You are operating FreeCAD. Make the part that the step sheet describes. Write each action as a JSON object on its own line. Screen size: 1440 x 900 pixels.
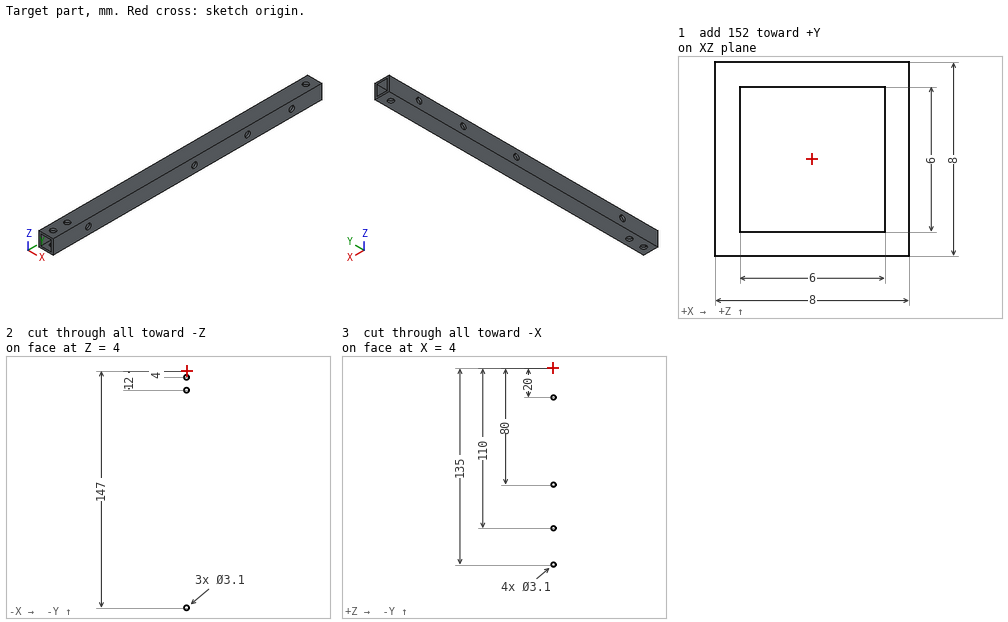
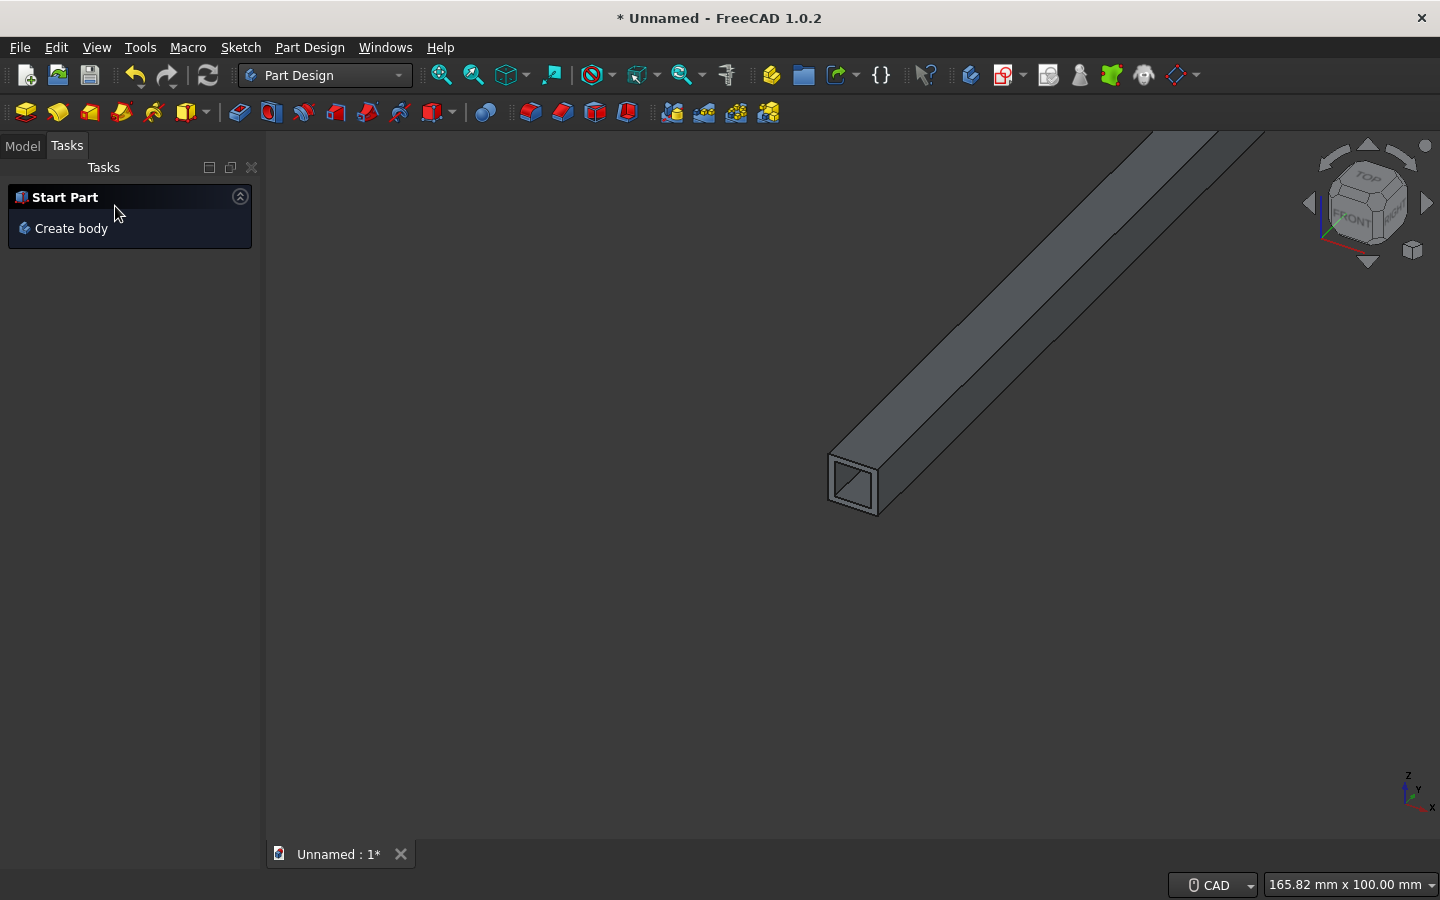
{"action": "left_click", "coordinate": [442, 76]}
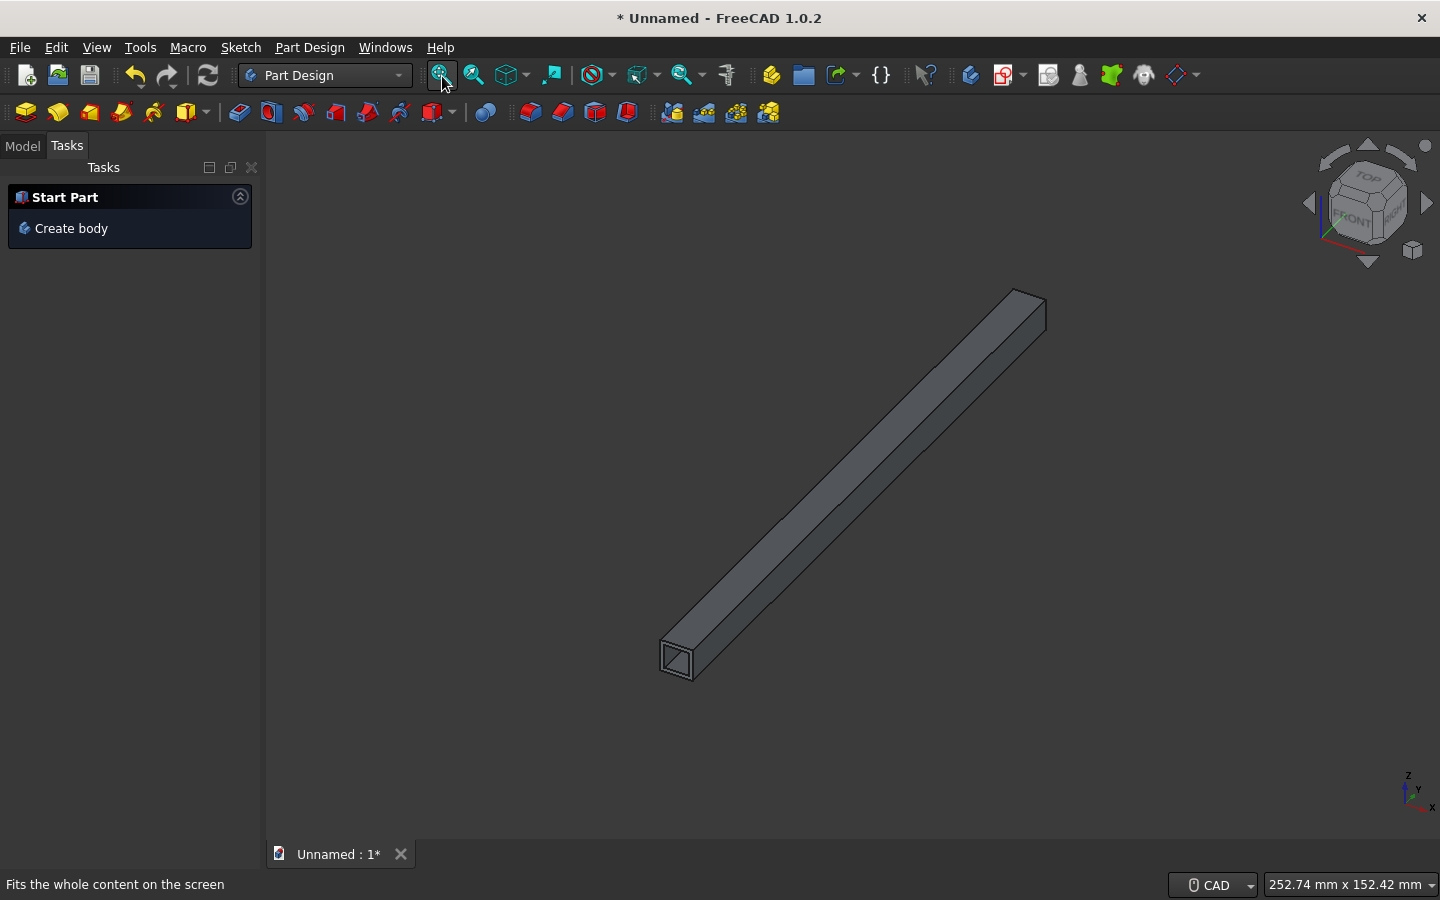
{"action": "left_click", "coordinate": [1004, 318]}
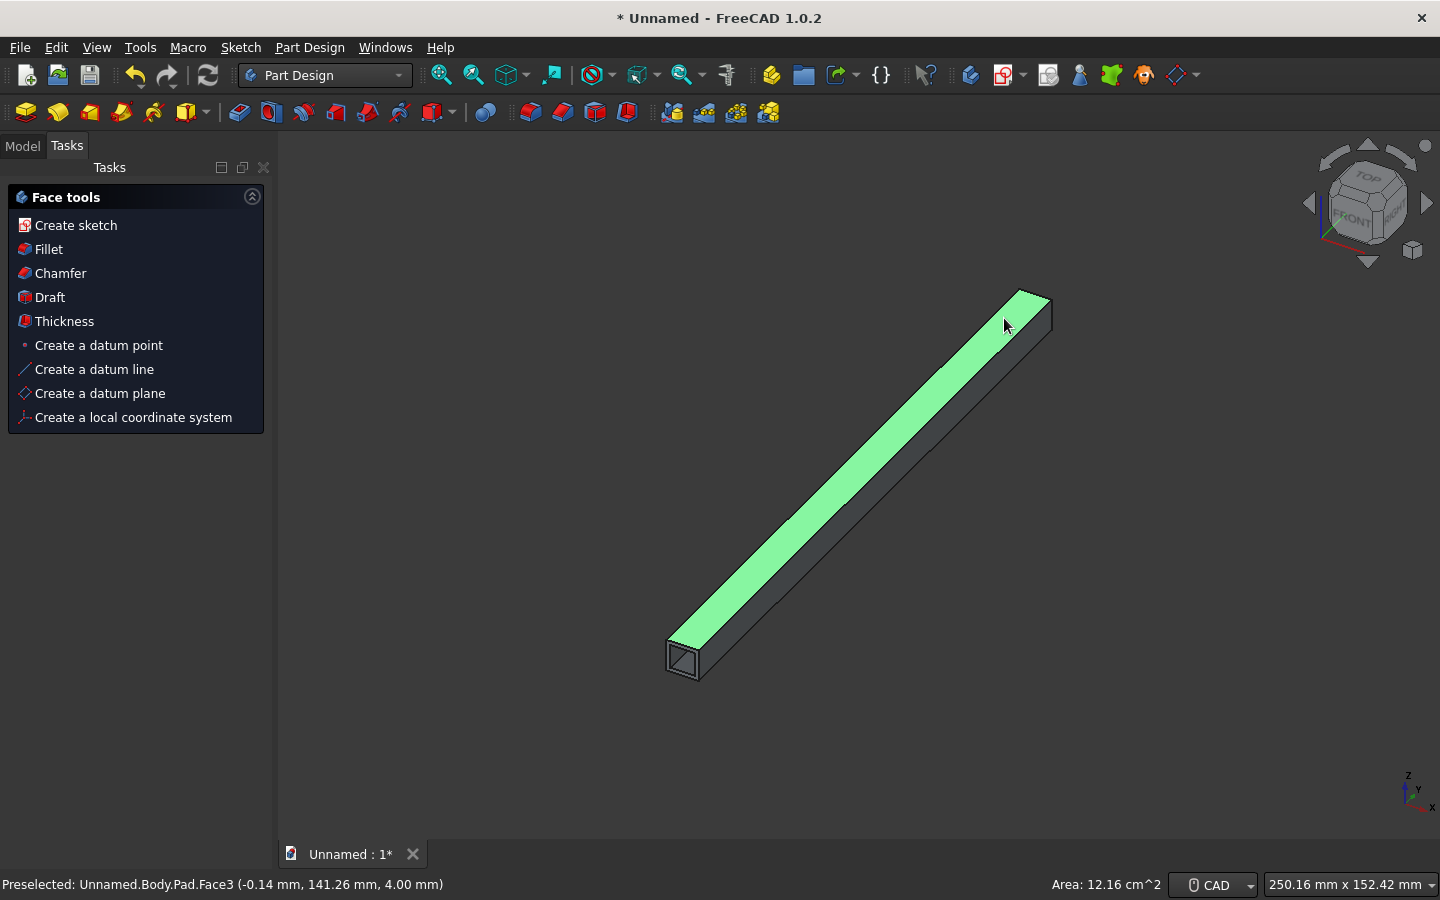
{"action": "left_click", "coordinate": [1004, 76]}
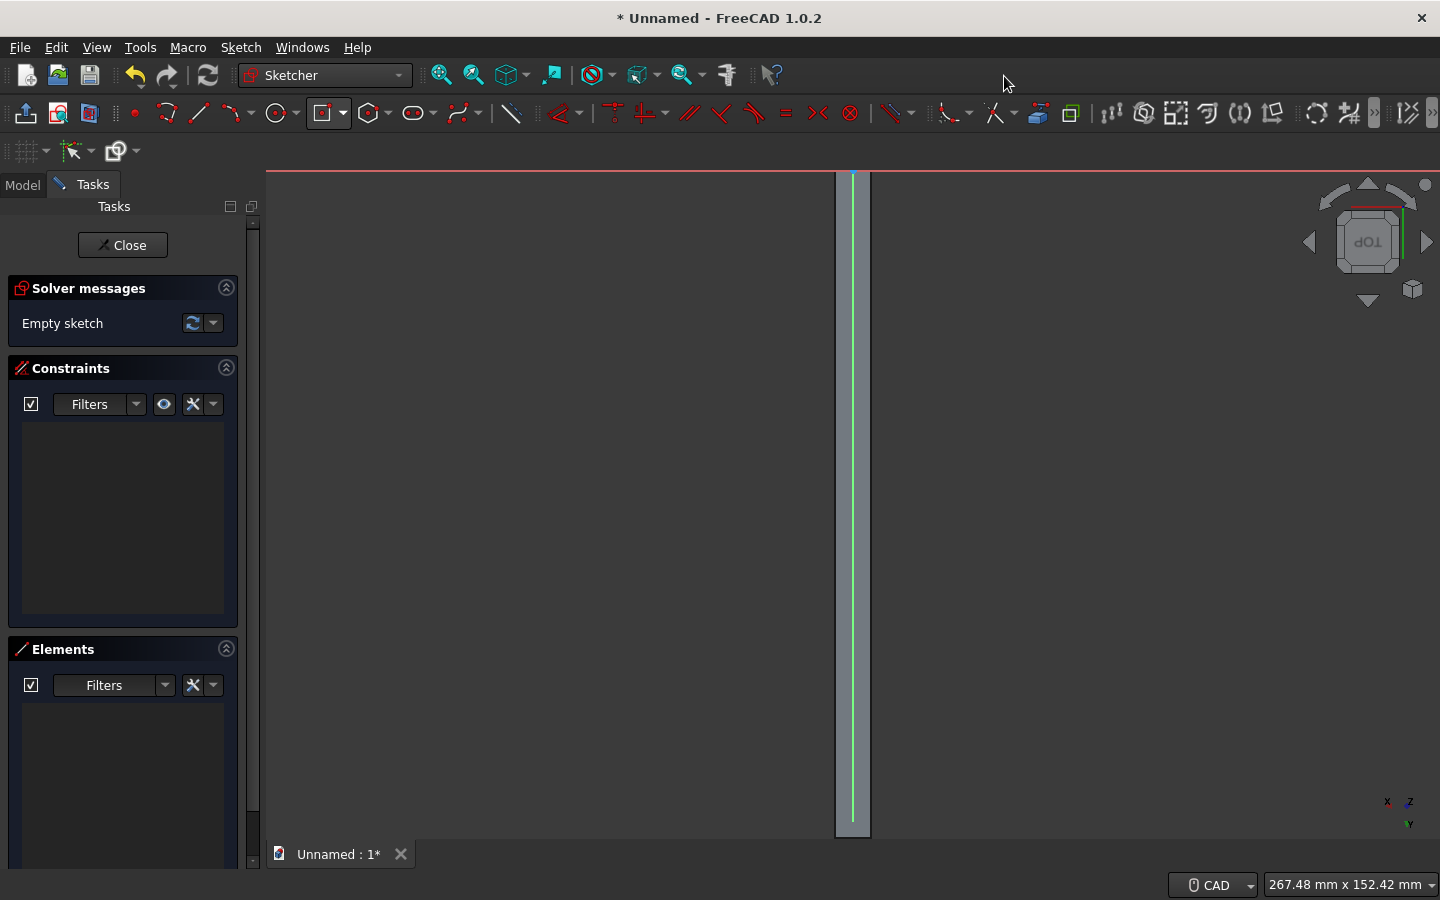
{"action": "scroll", "coordinate": [645, 520], "scroll_direction": "down", "scroll_amount": 2}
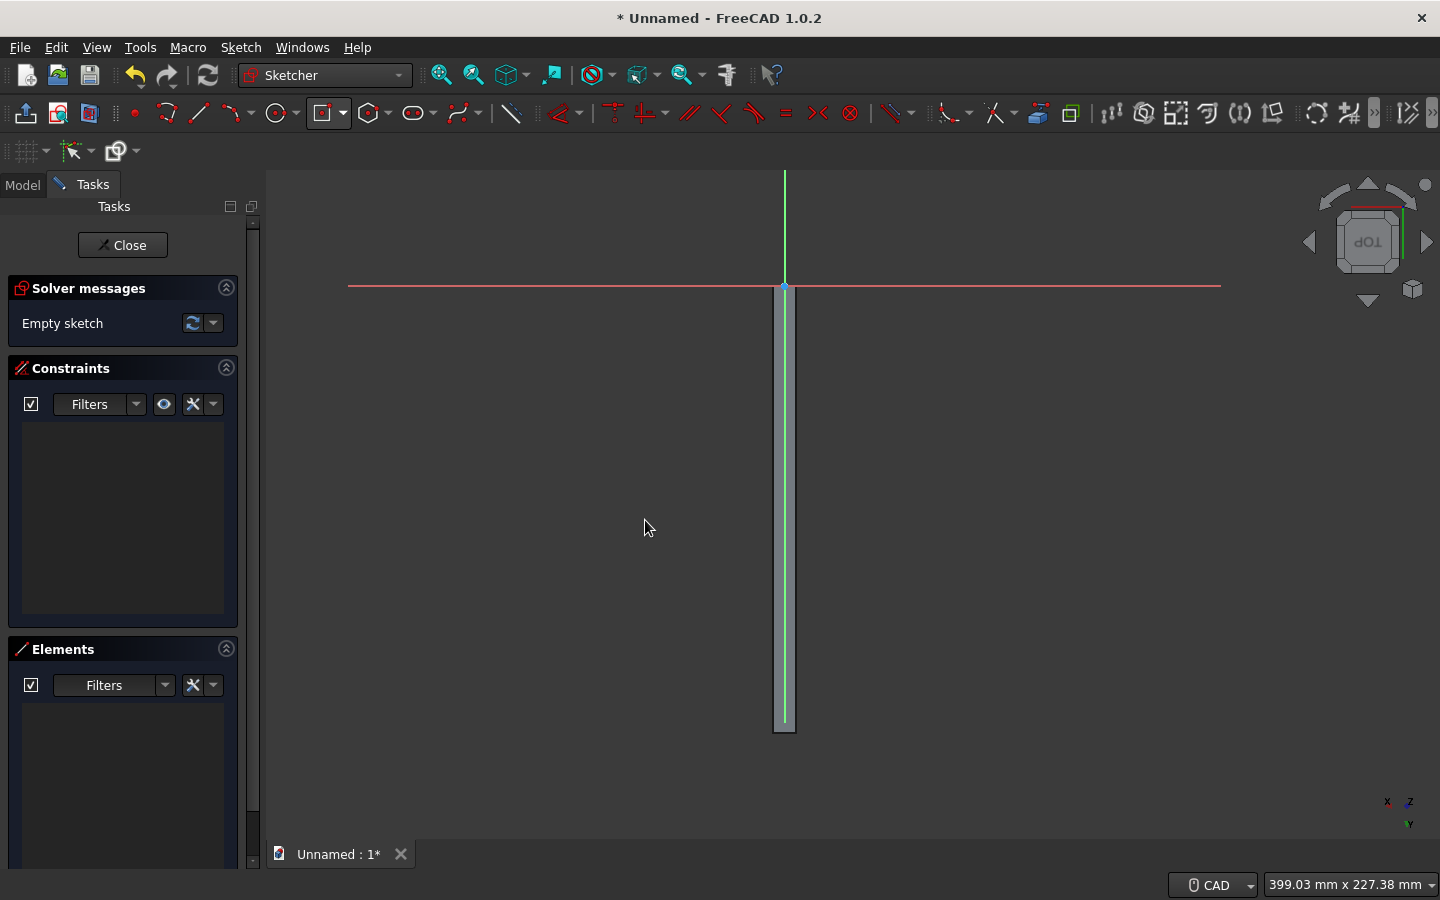
{"action": "left_click", "coordinate": [276, 114]}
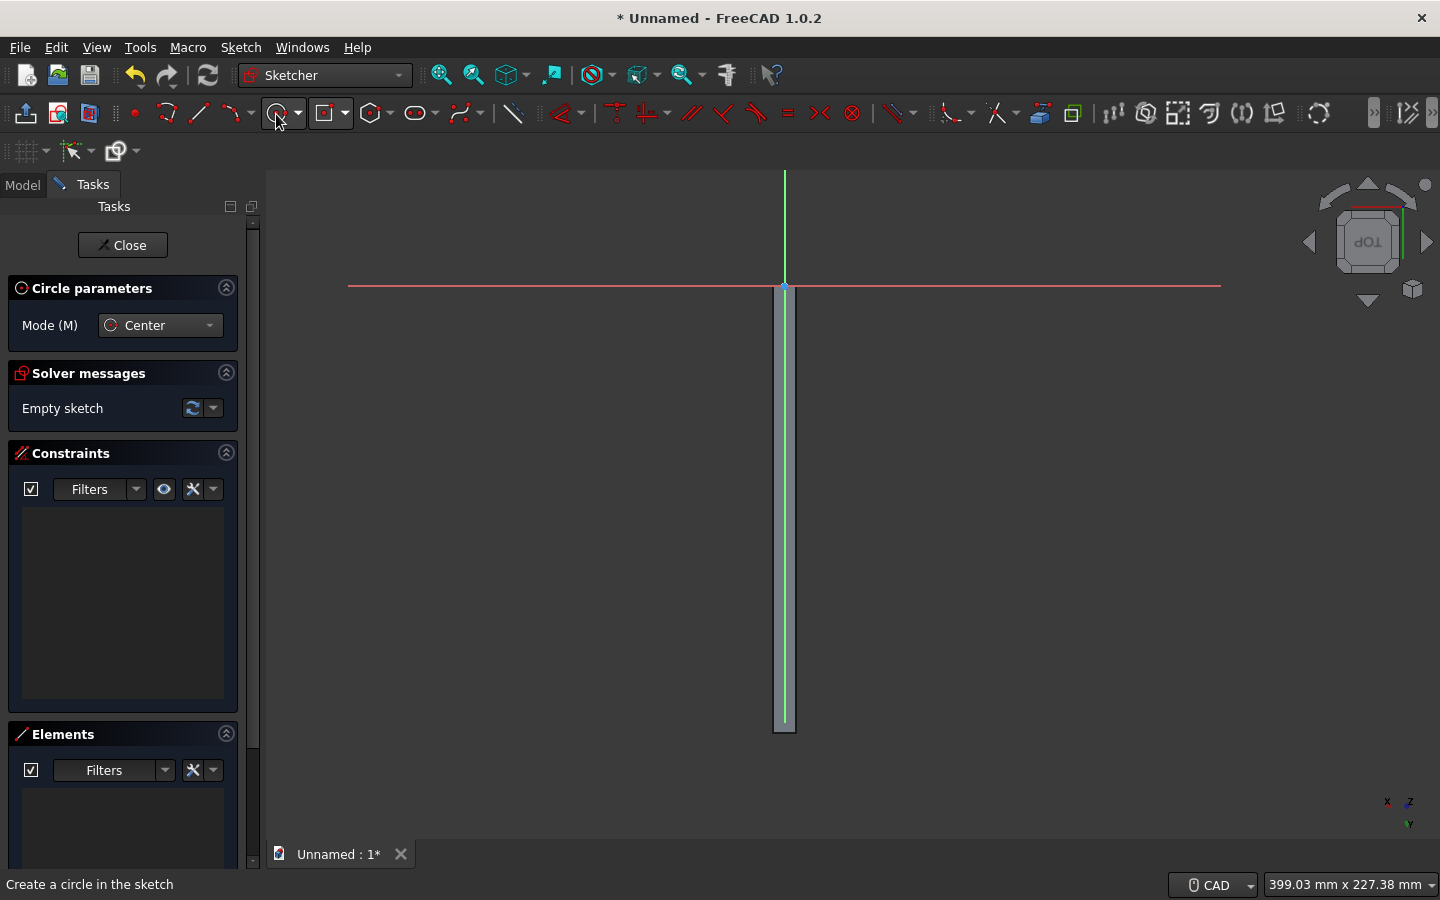
{"action": "scroll", "coordinate": [785, 719], "scroll_direction": "up", "scroll_amount": 9}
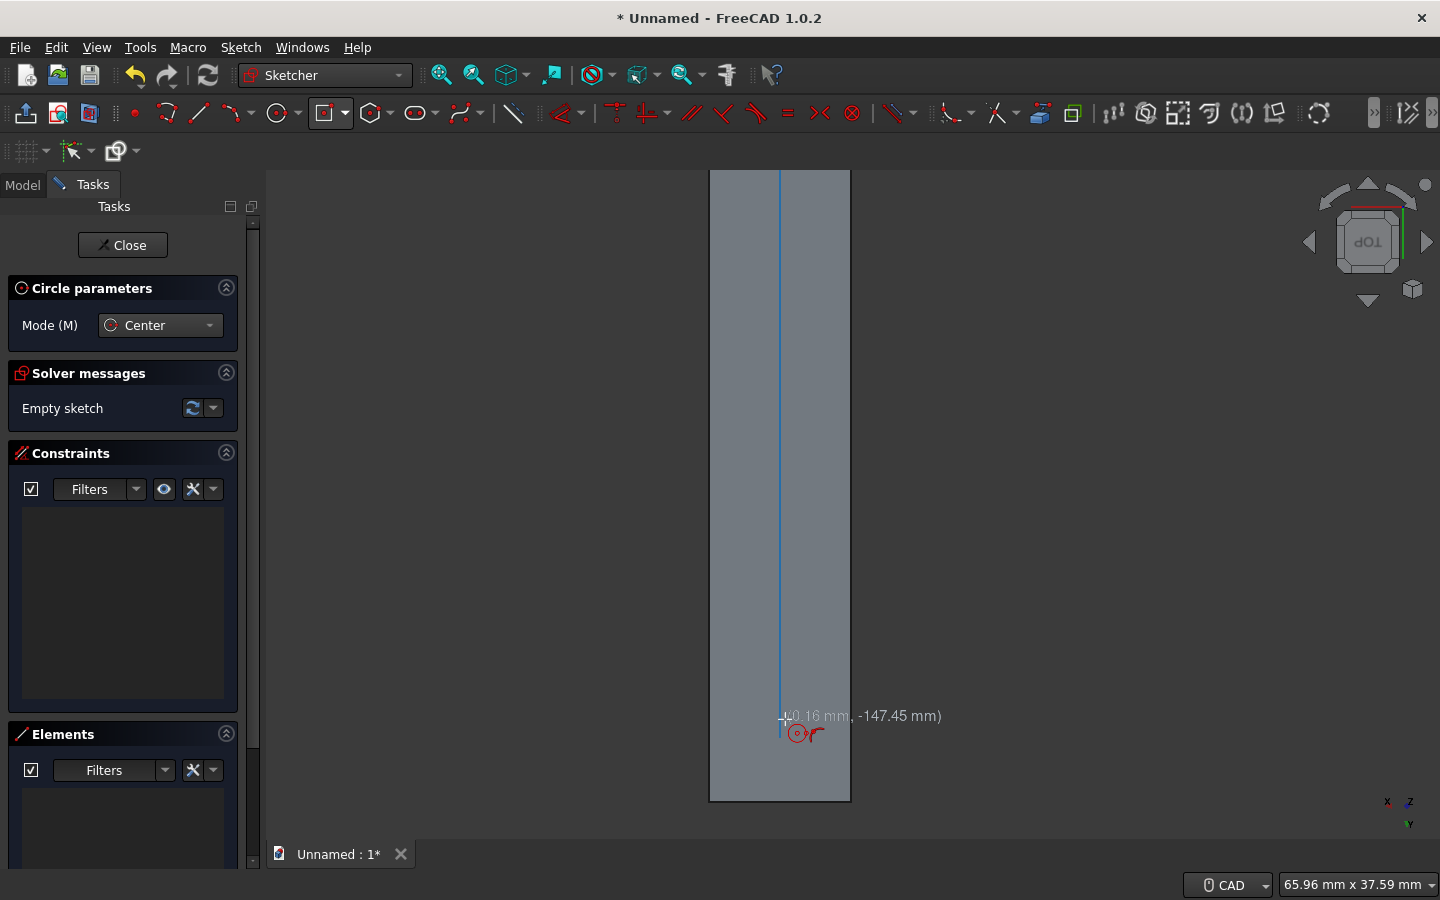
{"action": "scroll", "coordinate": [785, 720], "scroll_direction": "down", "scroll_amount": 9}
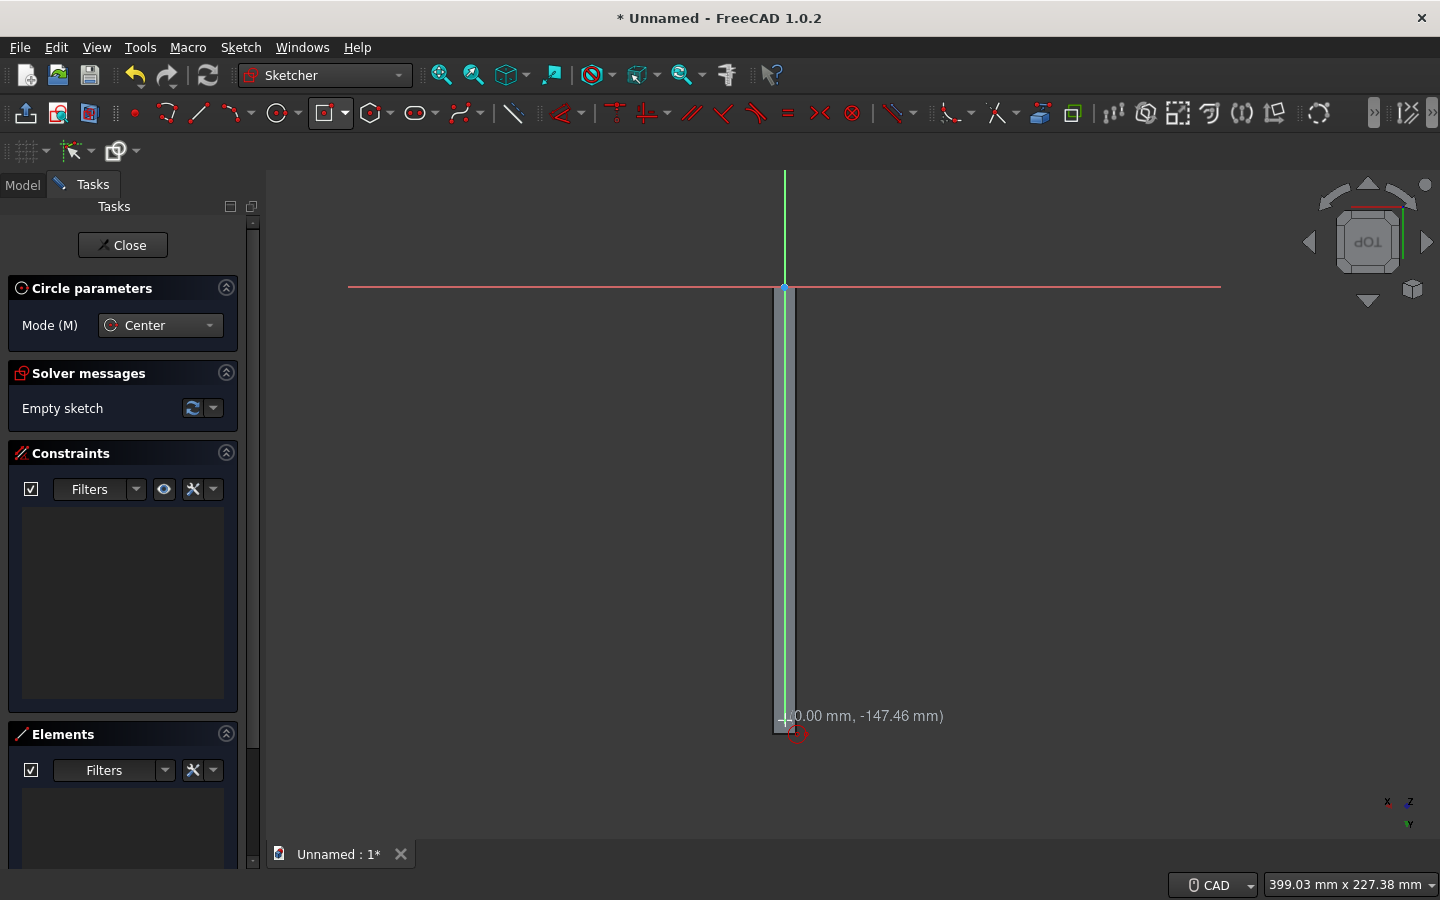
{"action": "left_click", "coordinate": [785, 720]}